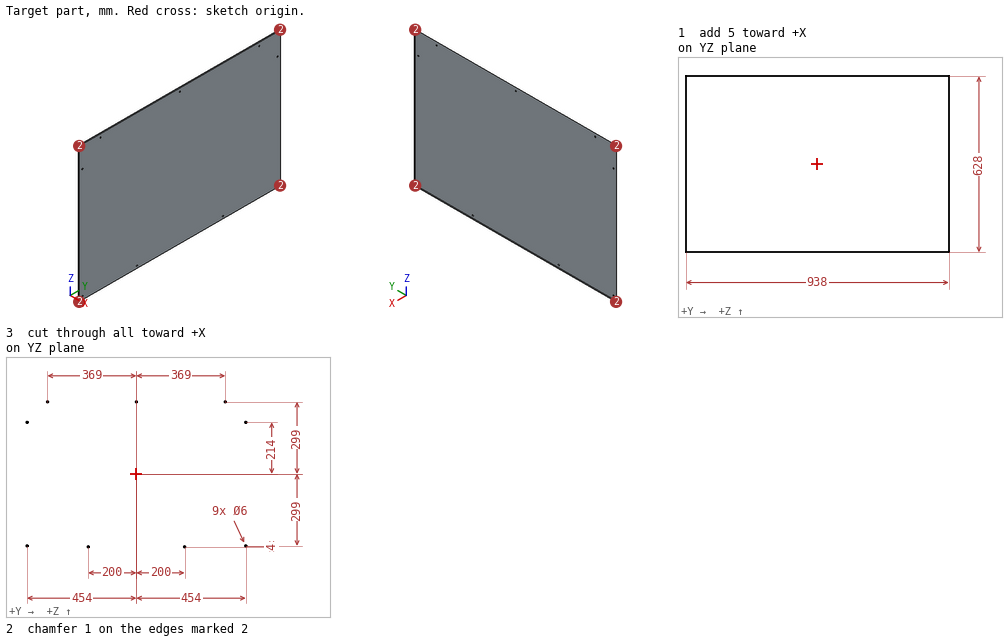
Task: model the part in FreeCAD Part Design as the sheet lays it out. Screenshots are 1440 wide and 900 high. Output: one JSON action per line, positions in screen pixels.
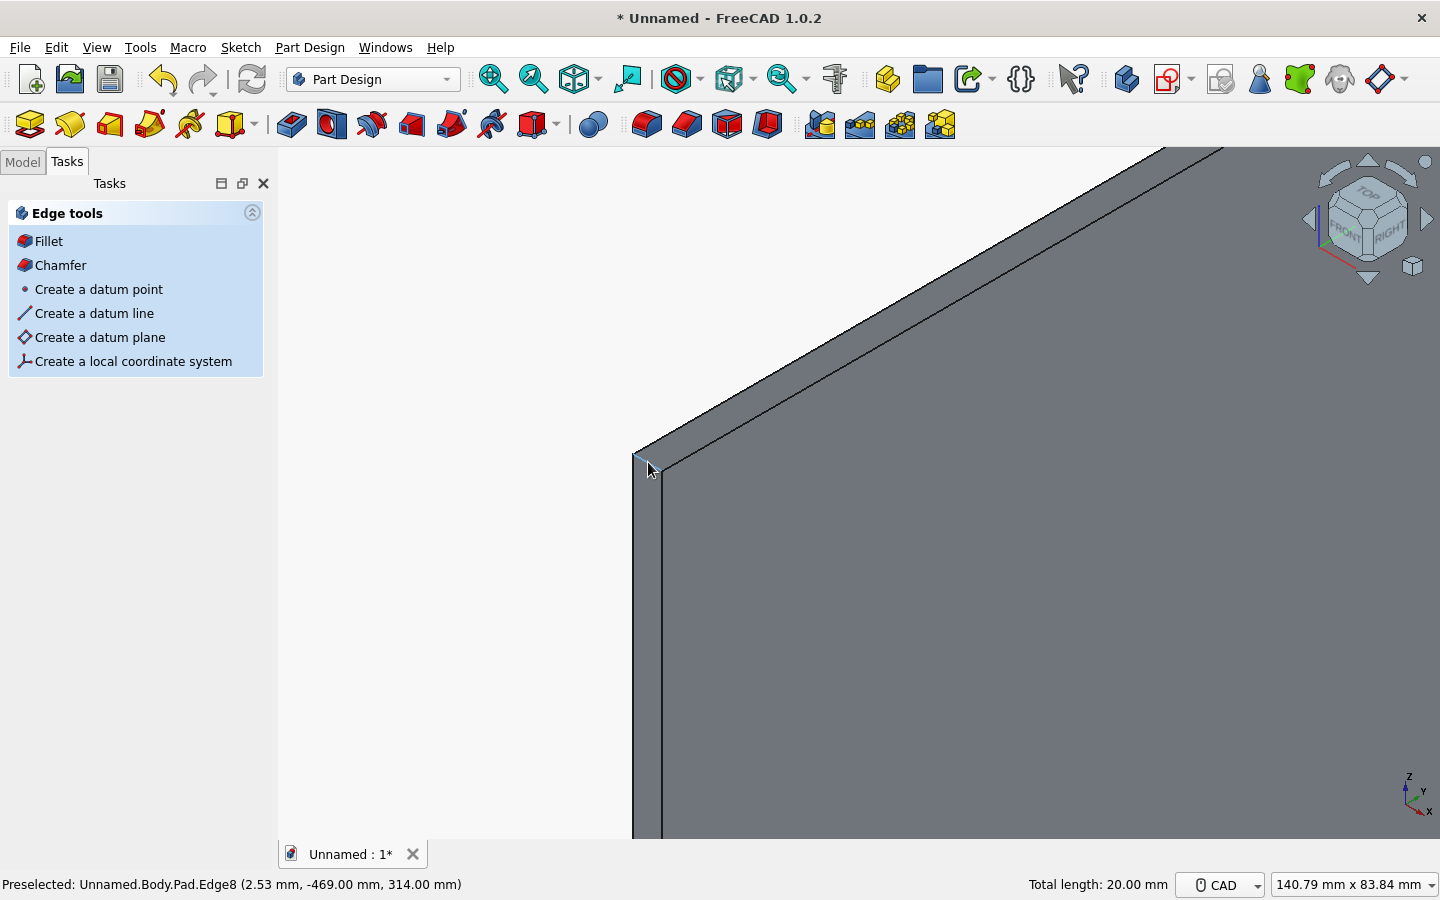
{"action": "left_click", "coordinate": [688, 124]}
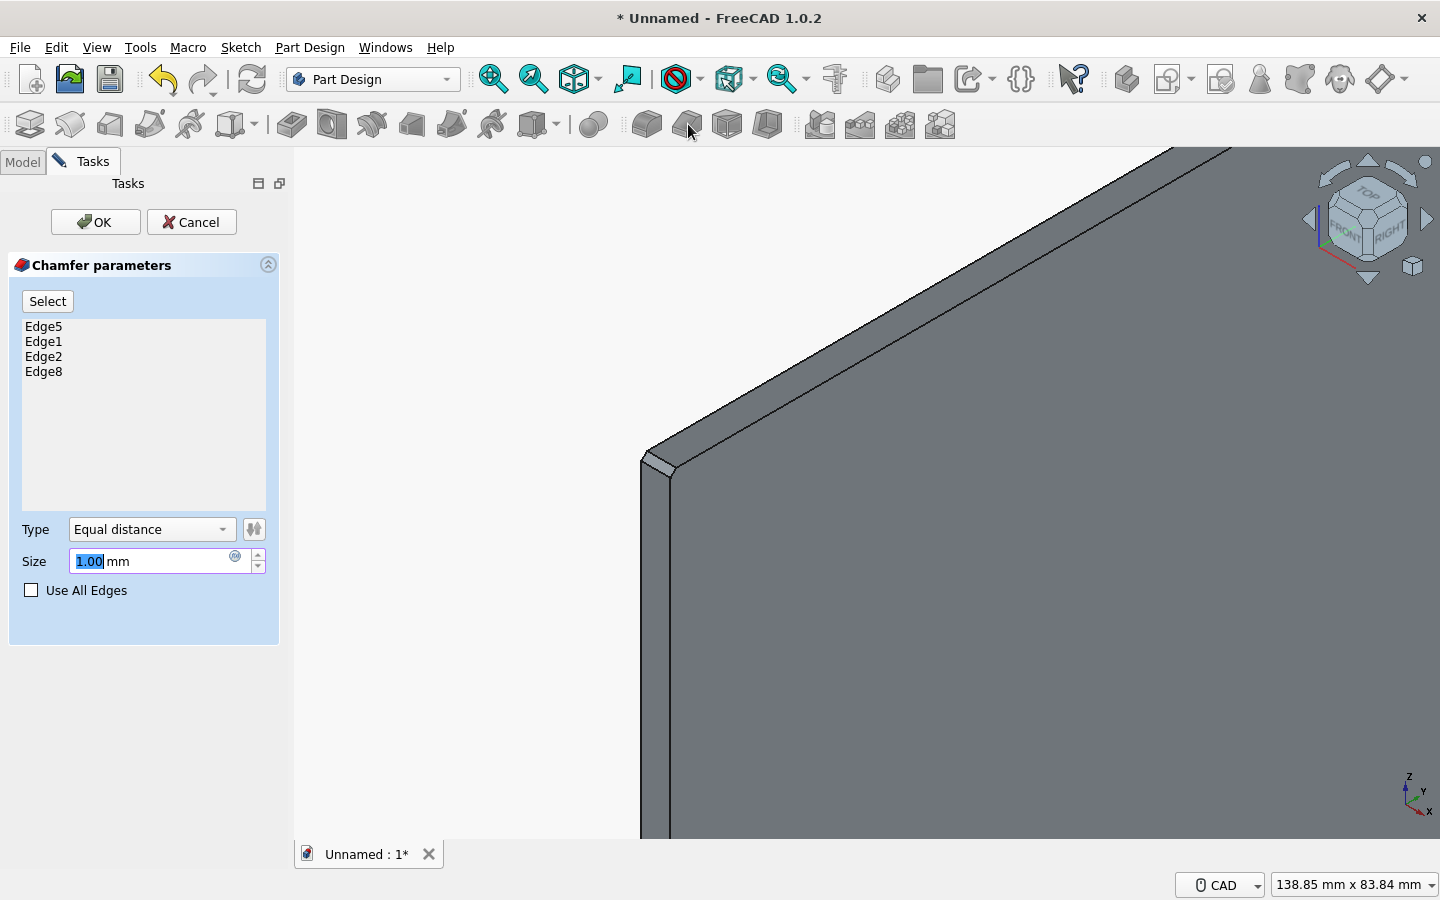
{"action": "type", "text": "1"}
{"action": "key", "text": "Tab"}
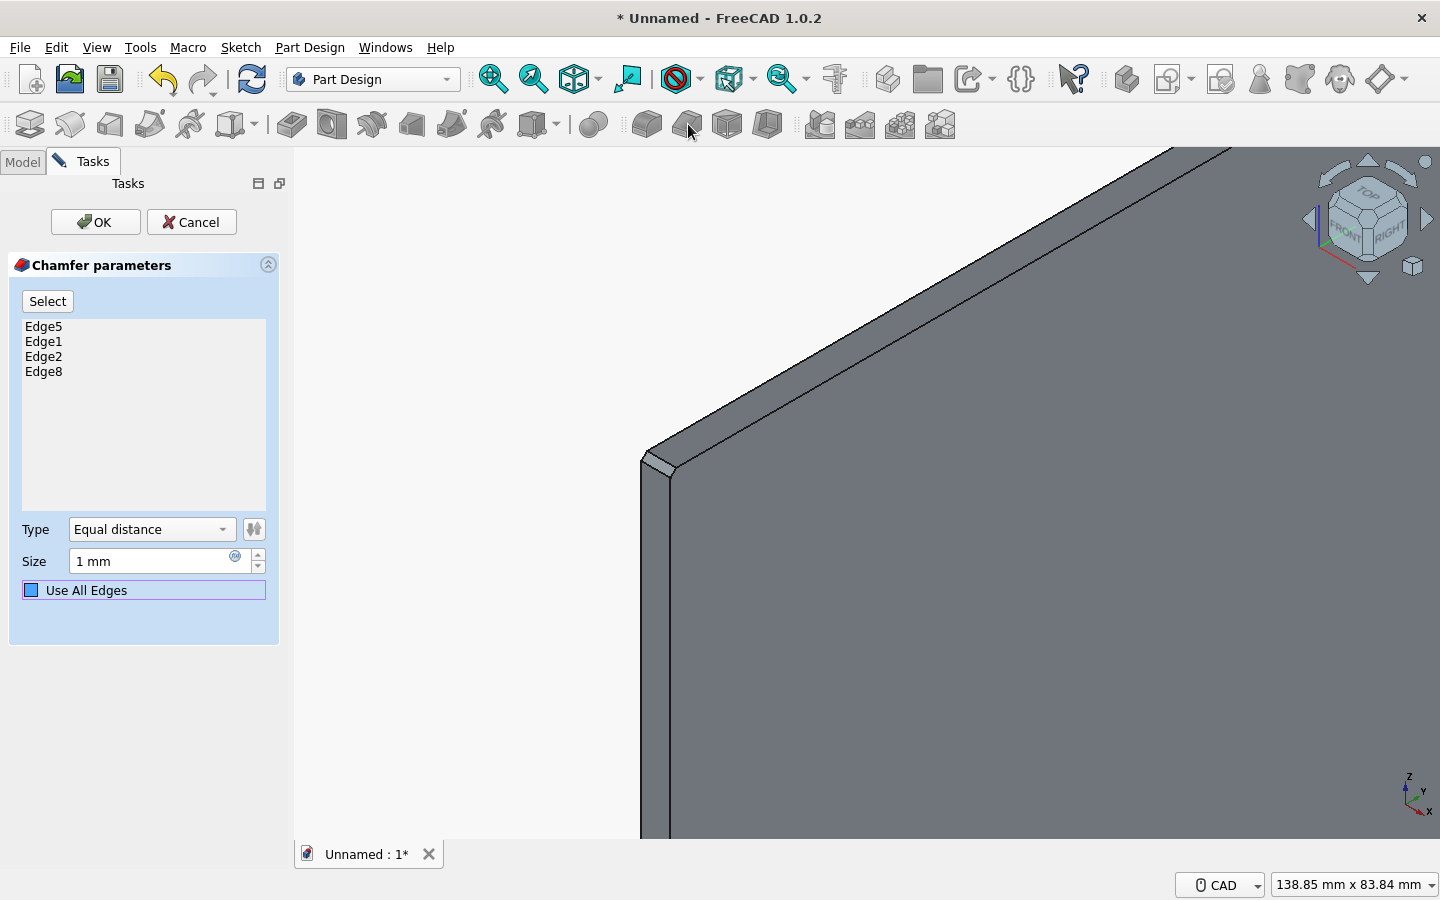
{"action": "left_click", "coordinate": [96, 222]}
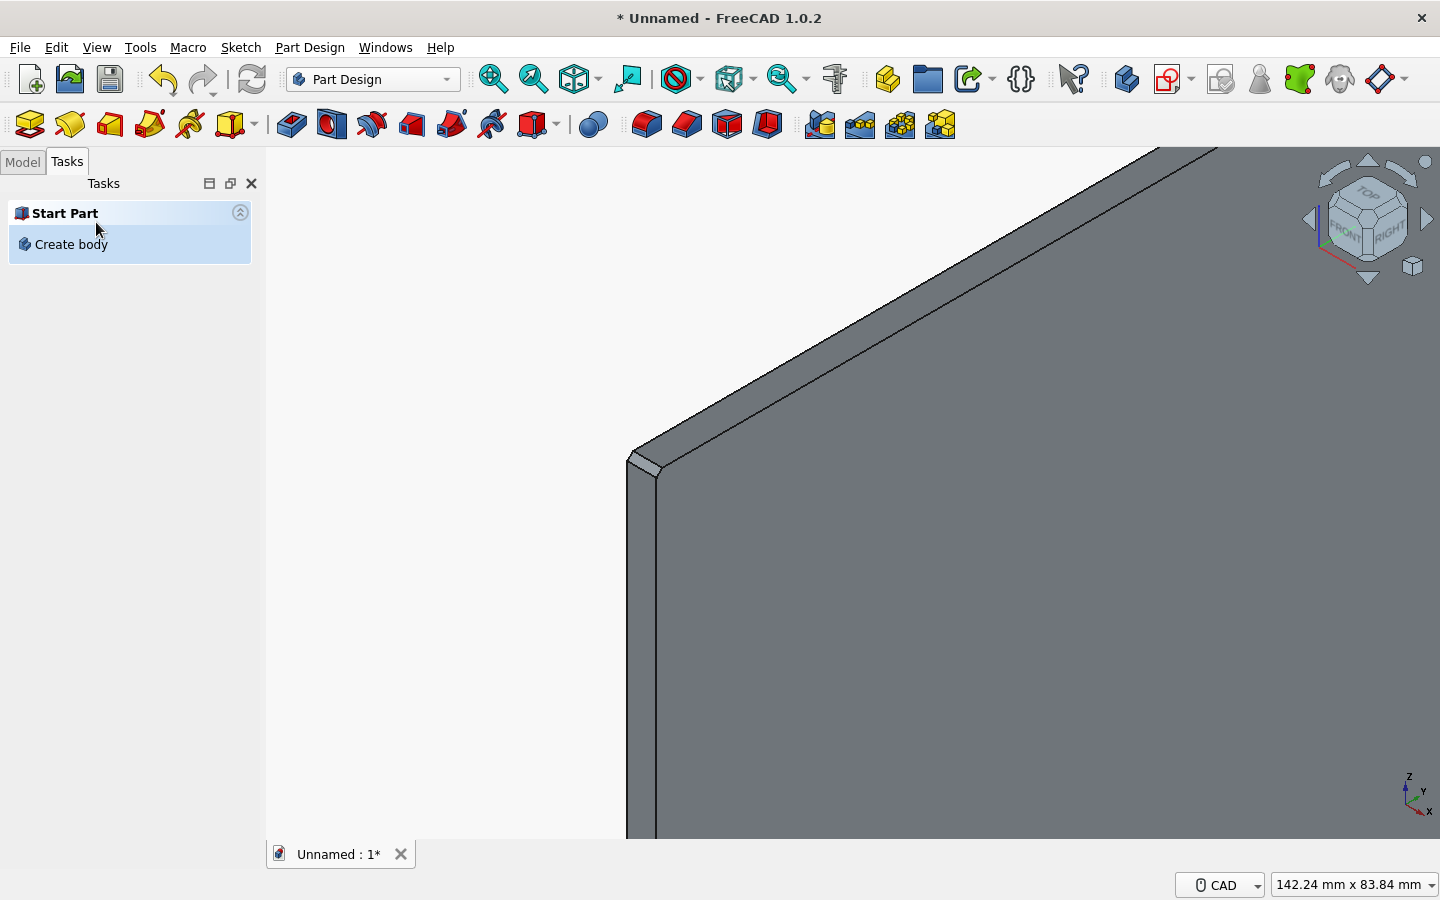
{"action": "key", "text": "v f"}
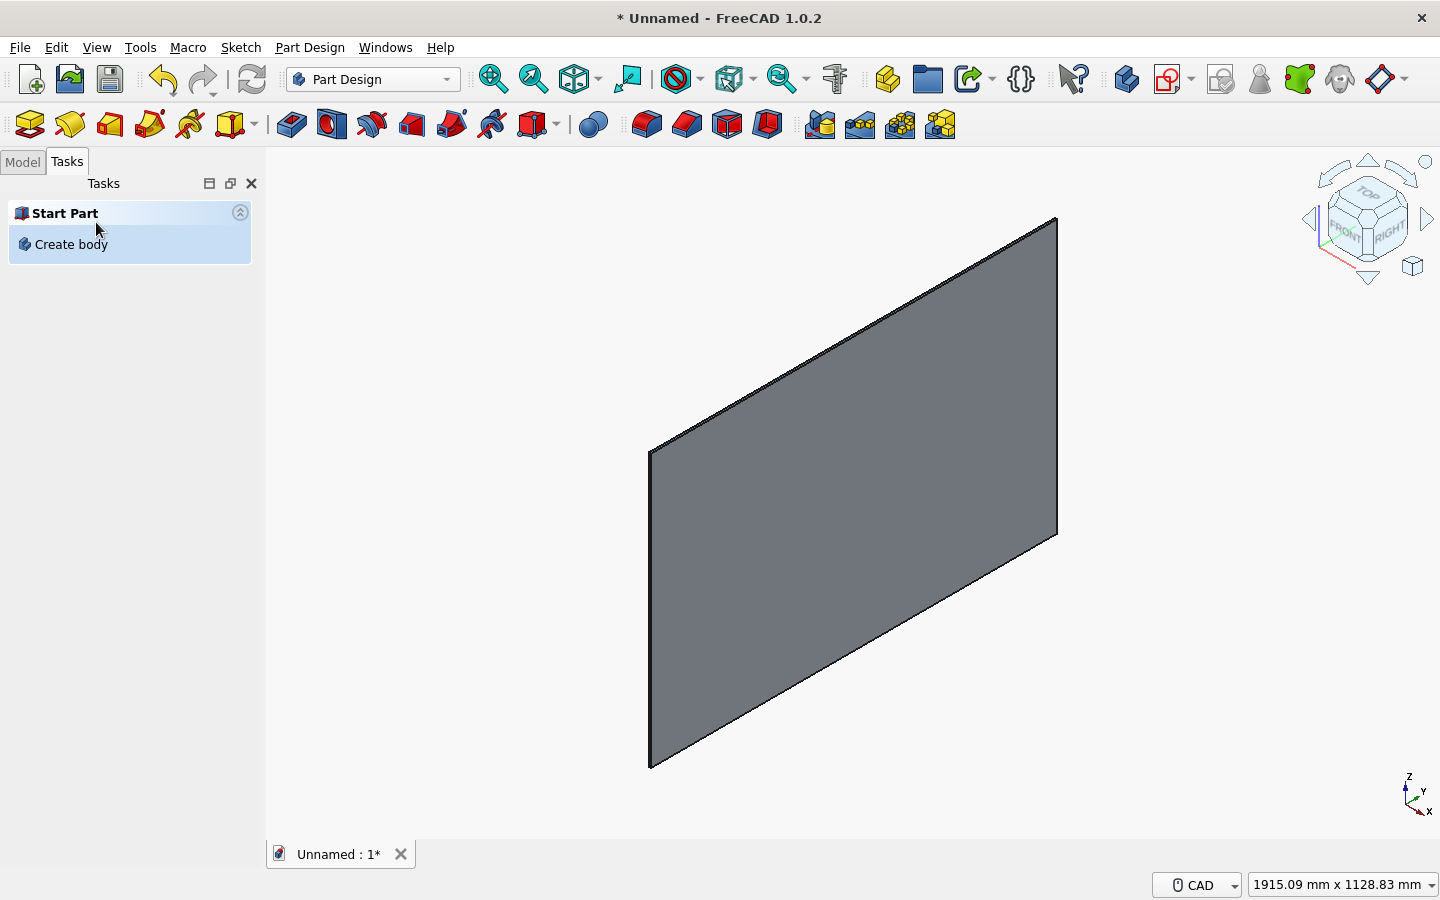
{"action": "left_click", "coordinate": [1168, 80]}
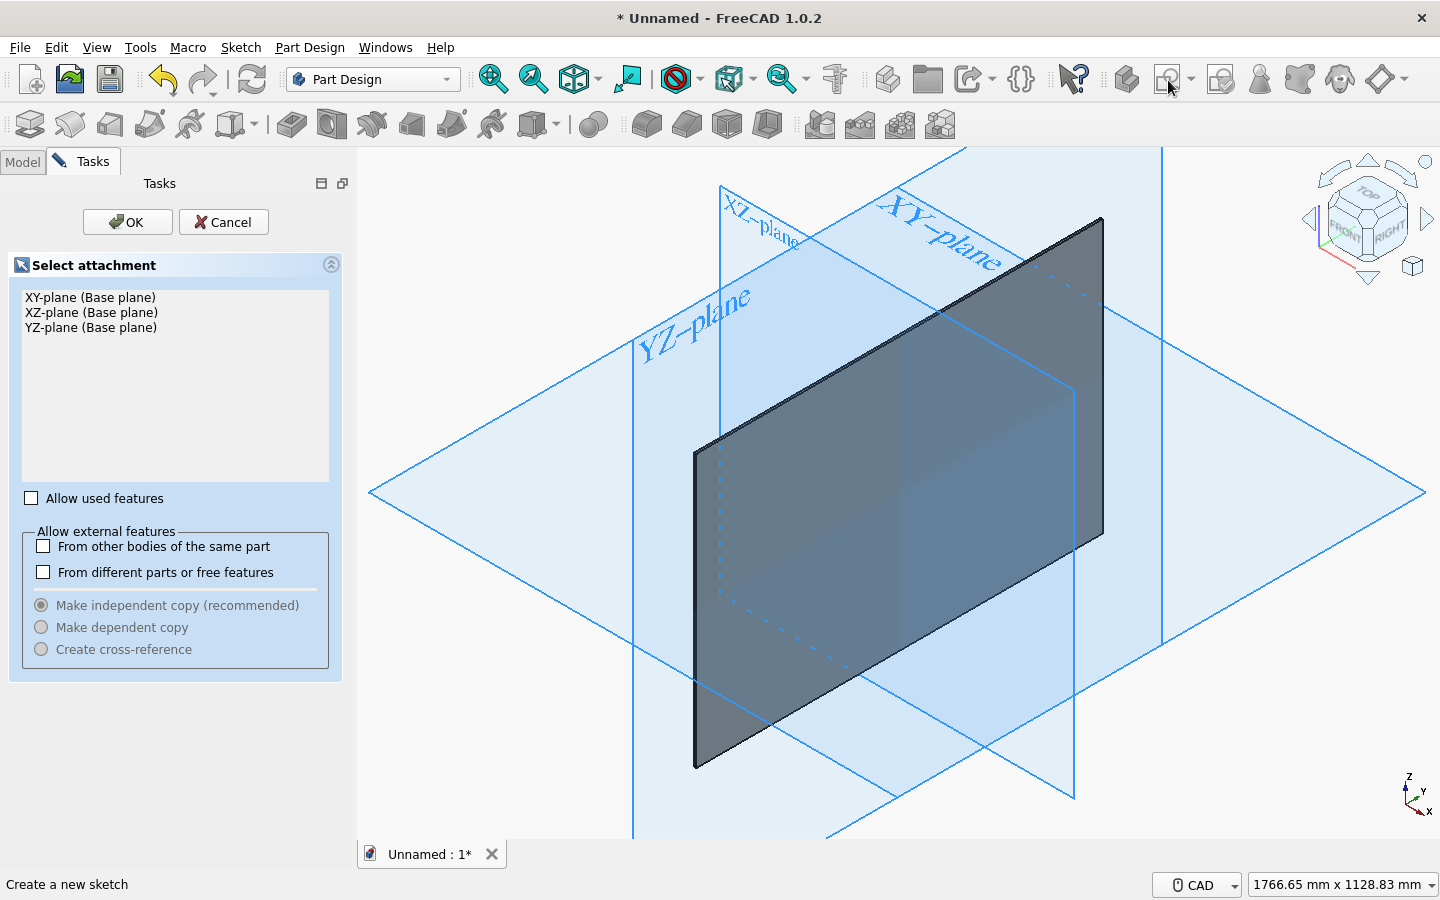
{"action": "left_click", "coordinate": [82, 328]}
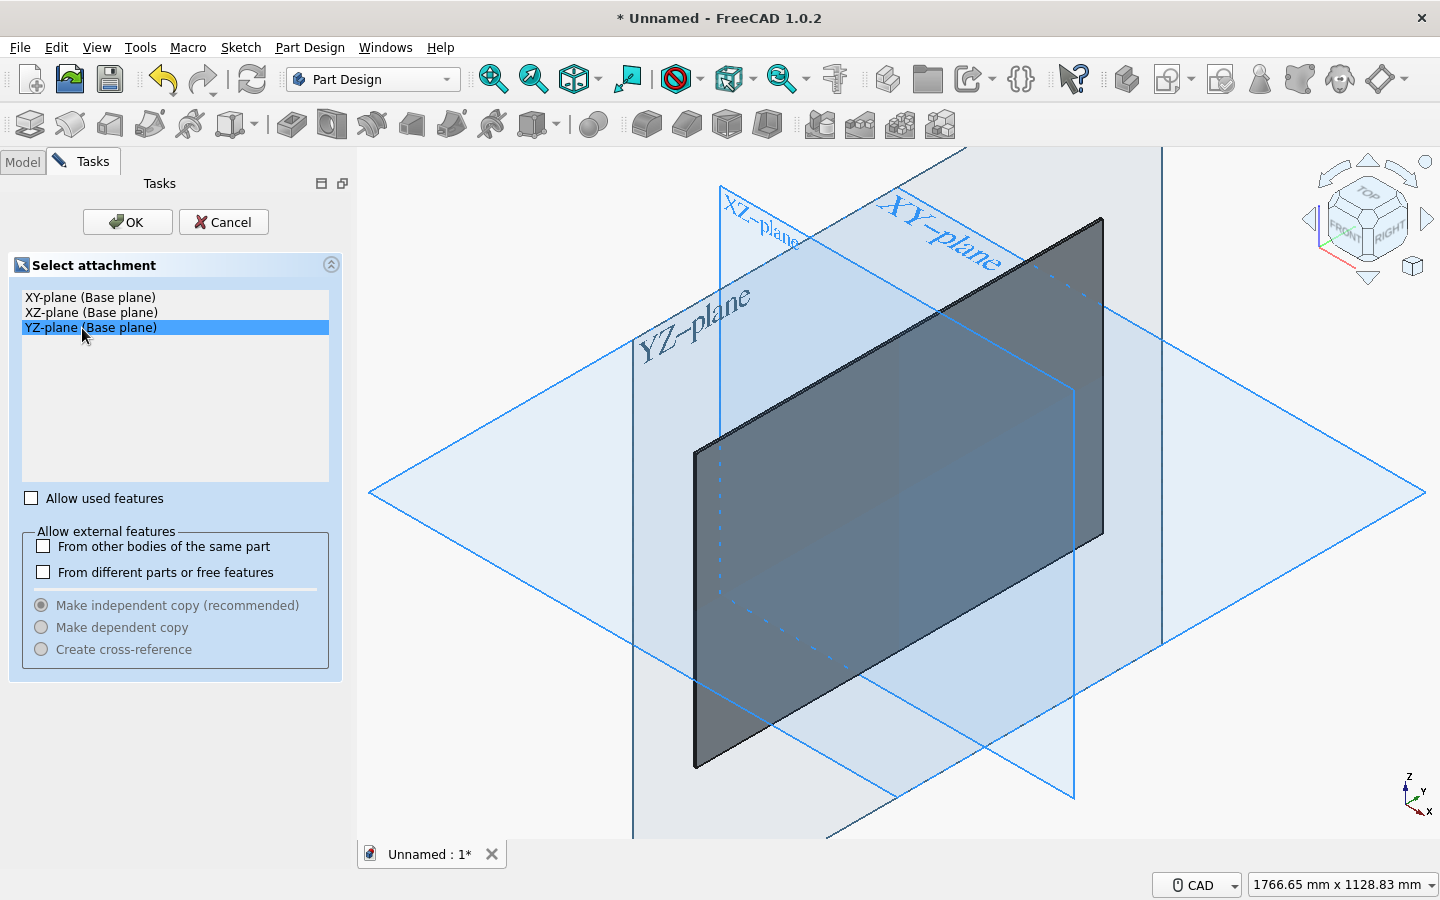
{"action": "left_click", "coordinate": [128, 222]}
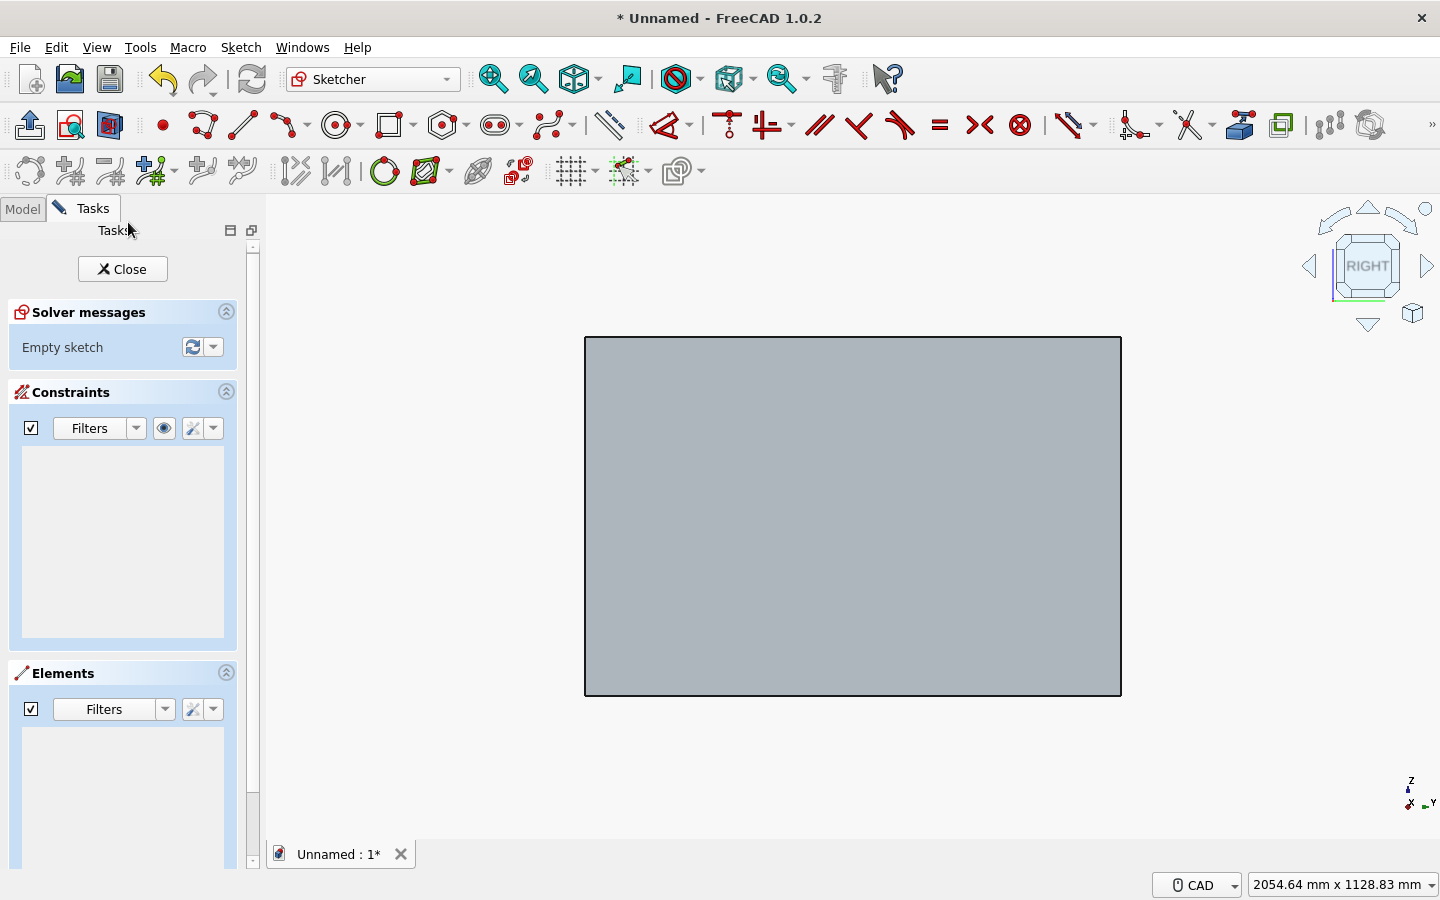
{"action": "key", "text": "q s"}